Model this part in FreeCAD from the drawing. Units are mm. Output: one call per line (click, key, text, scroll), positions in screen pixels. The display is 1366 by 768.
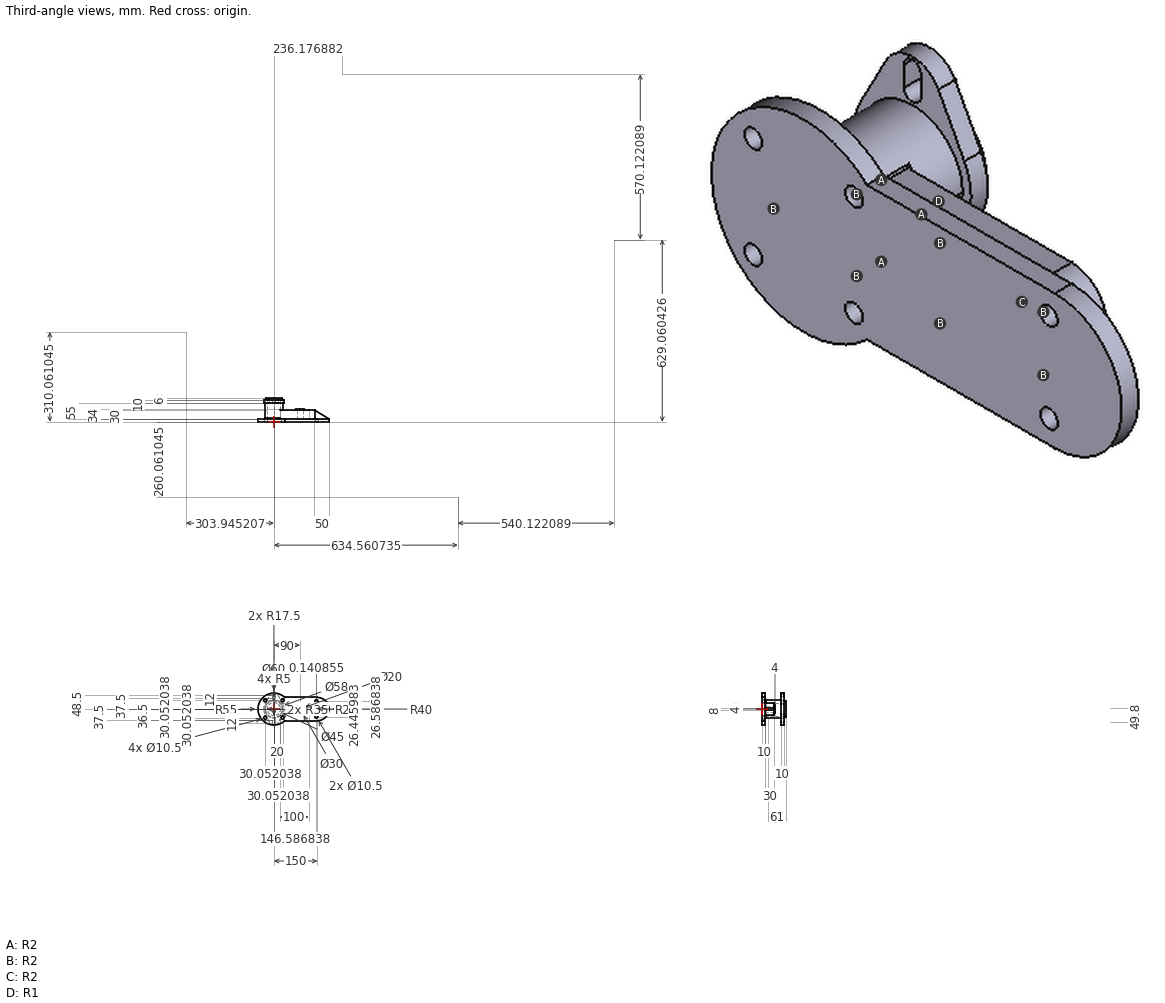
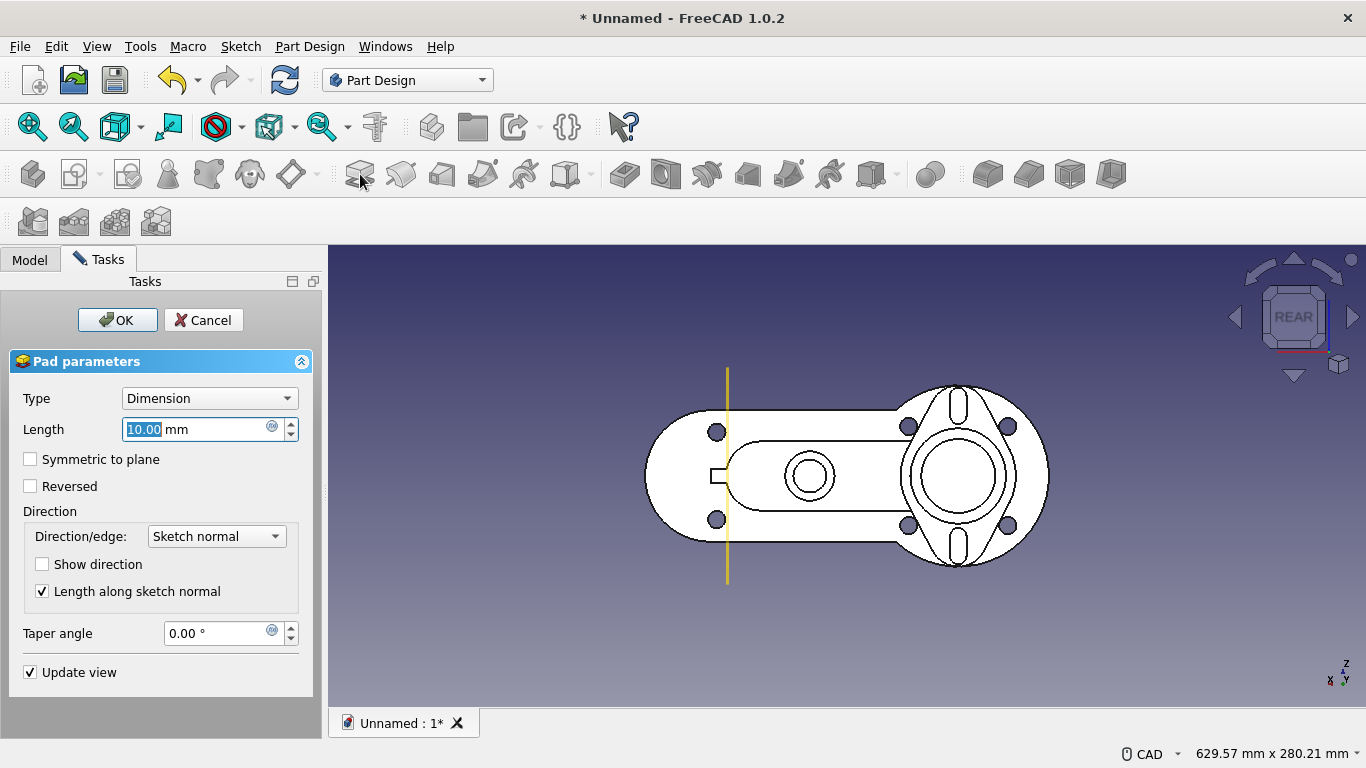
text(50)
key(Tab)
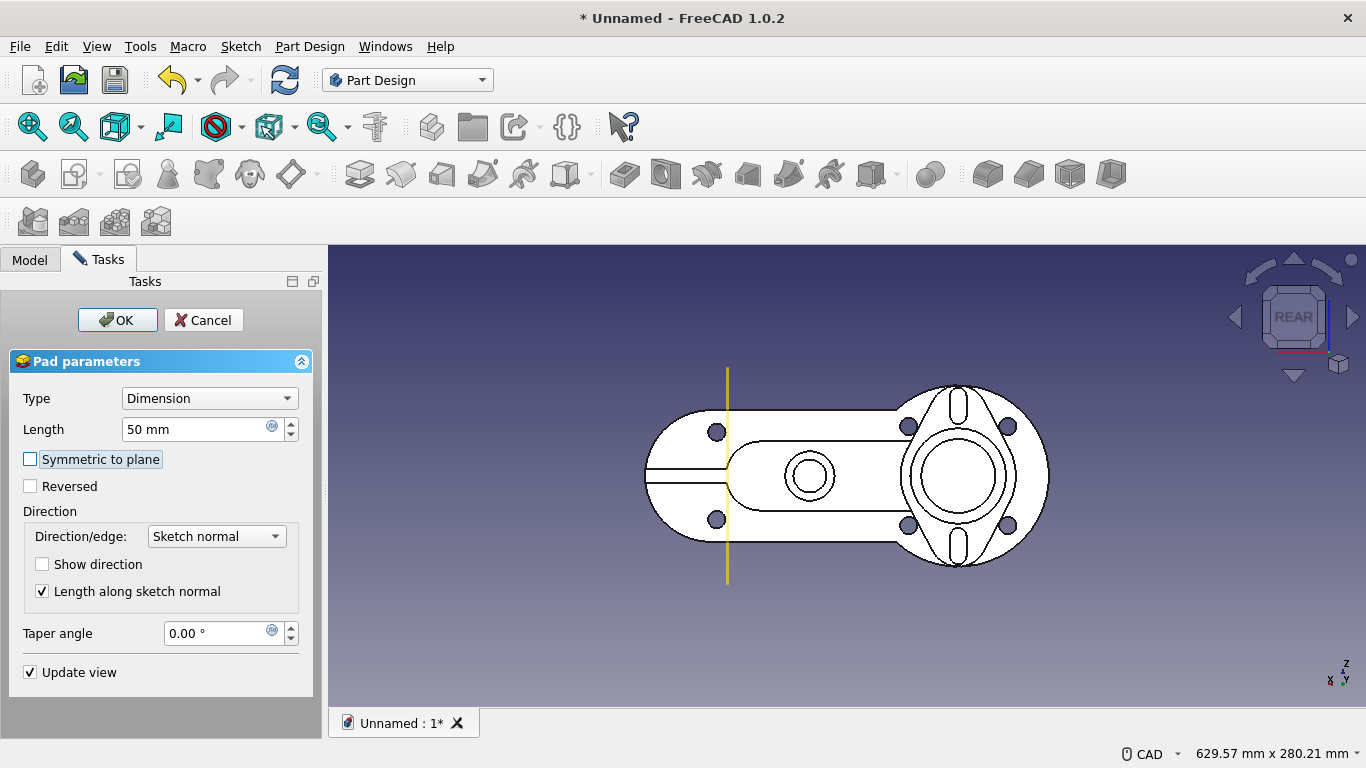
click(118, 320)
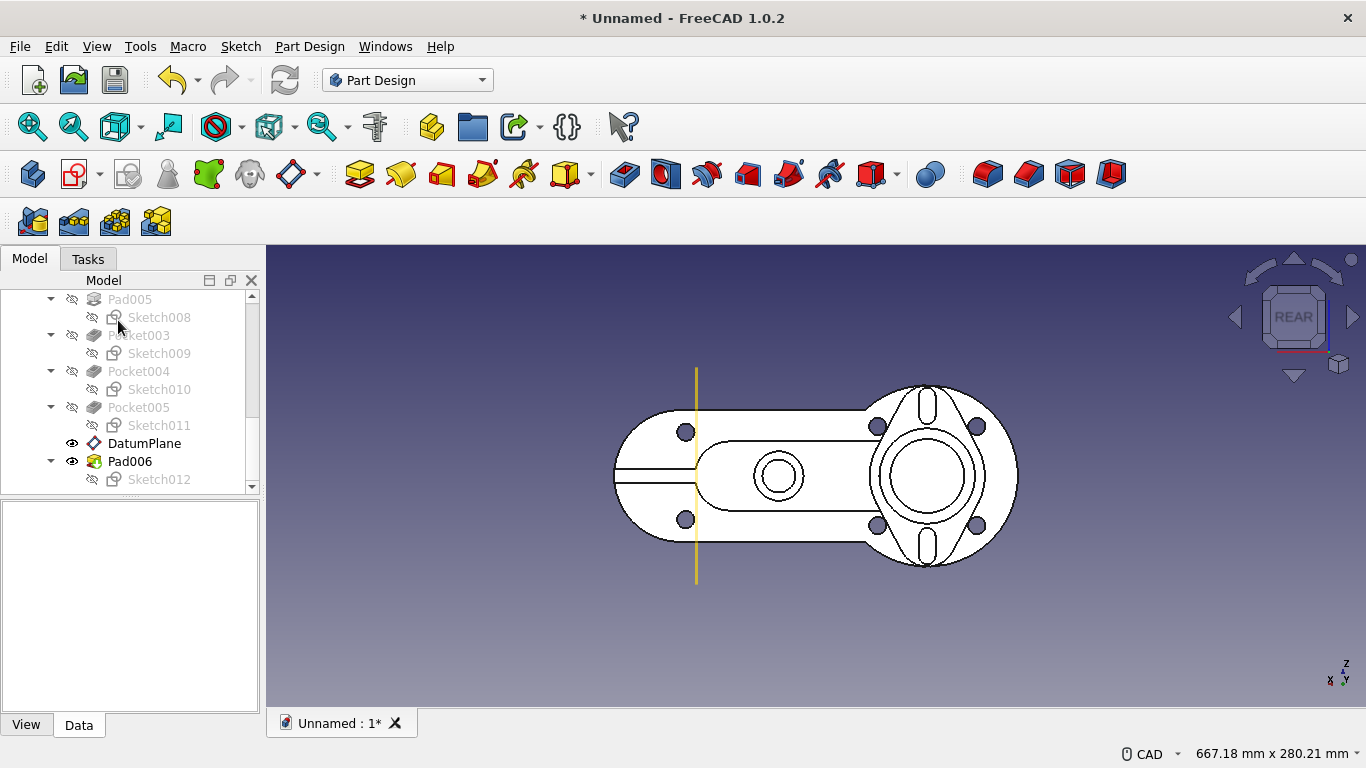
click(117, 443)
key(space)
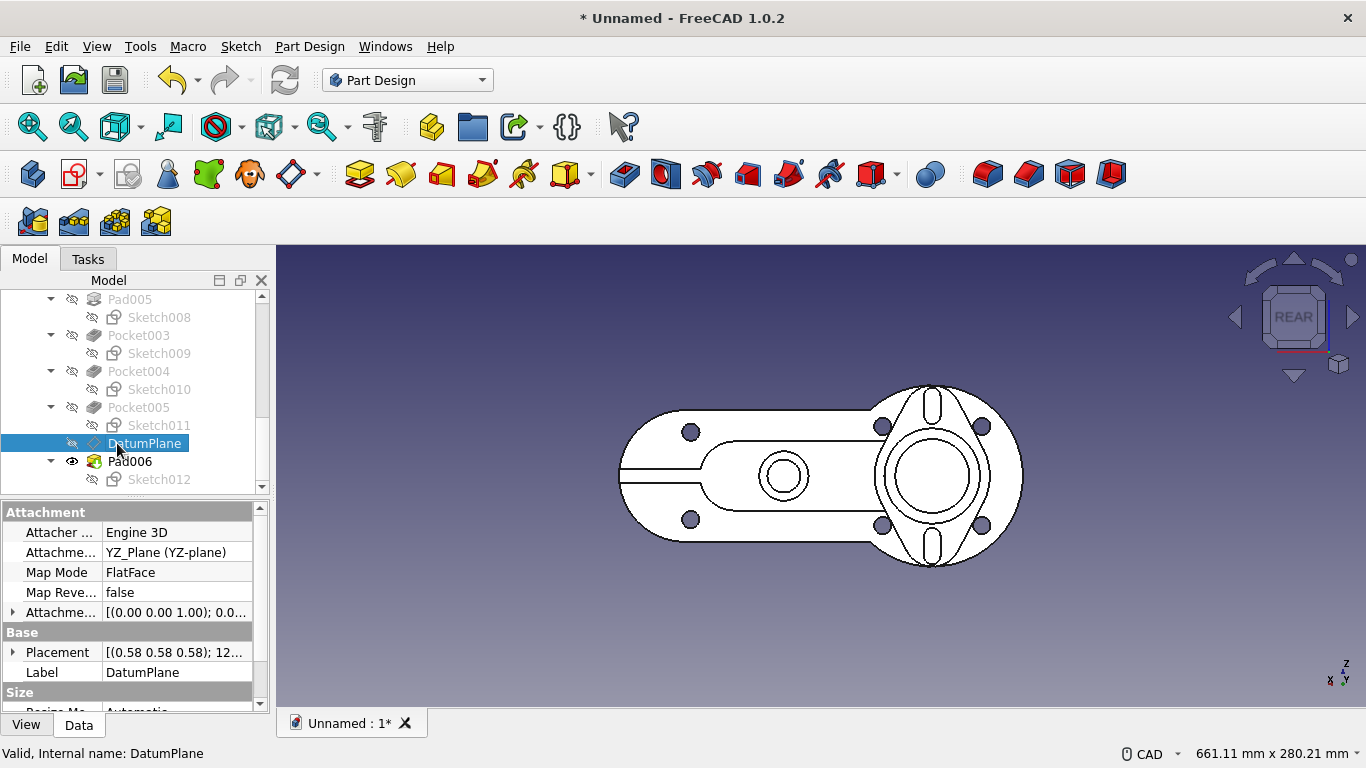
click(33, 128)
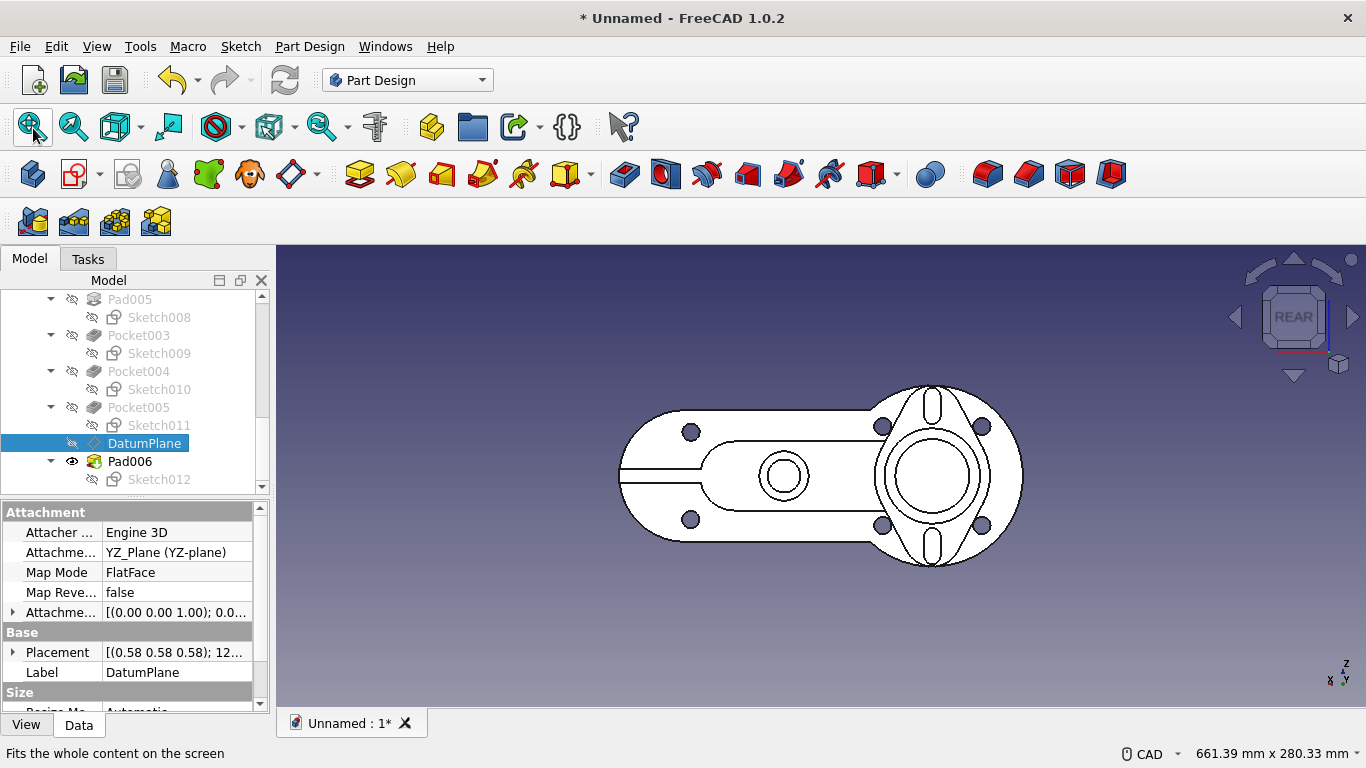
key(0)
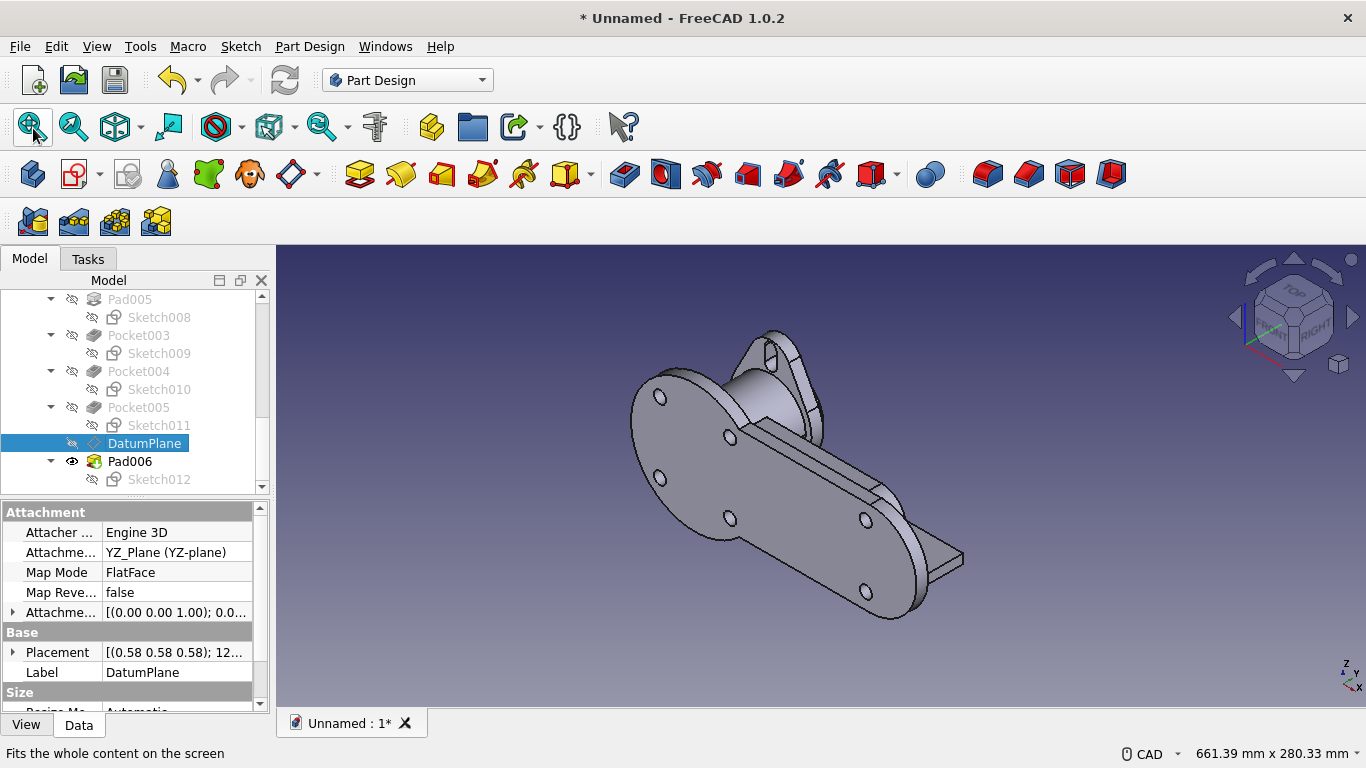
key(2)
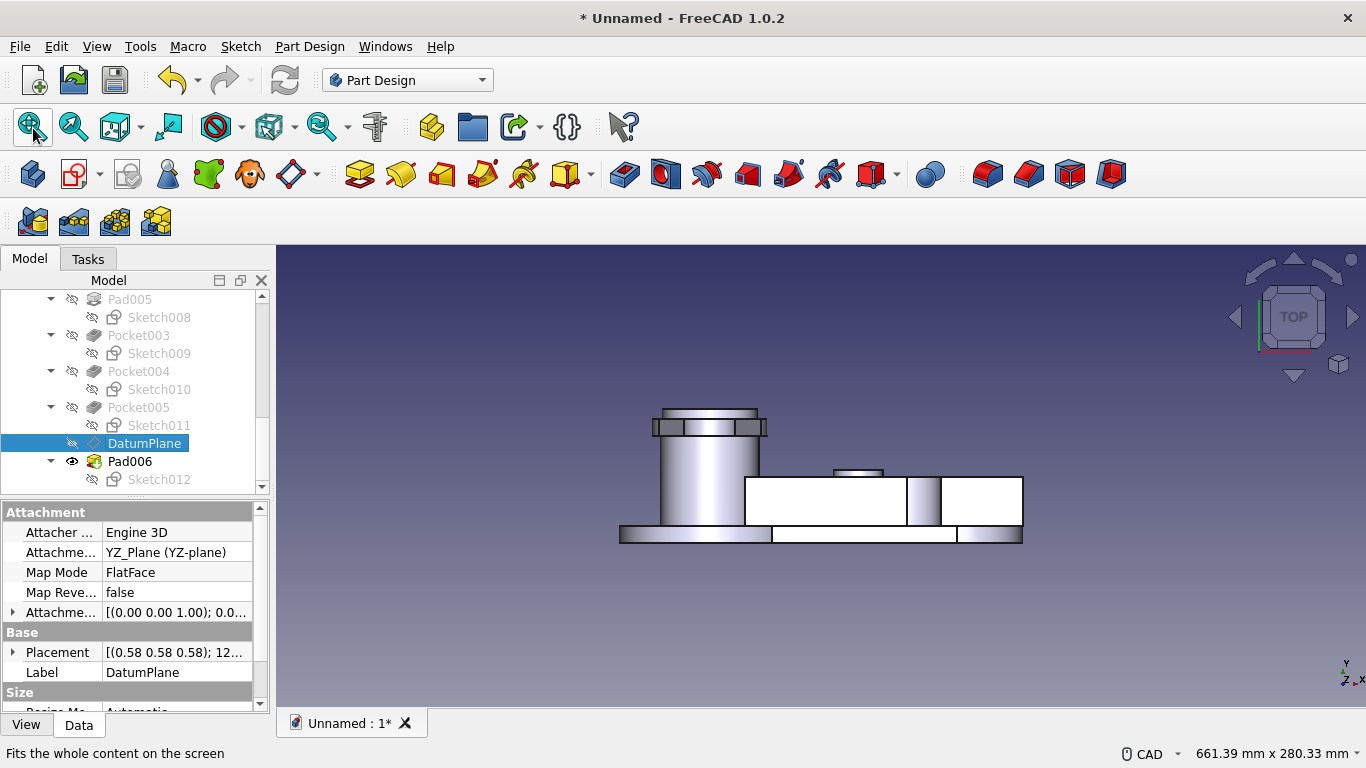
click(33, 128)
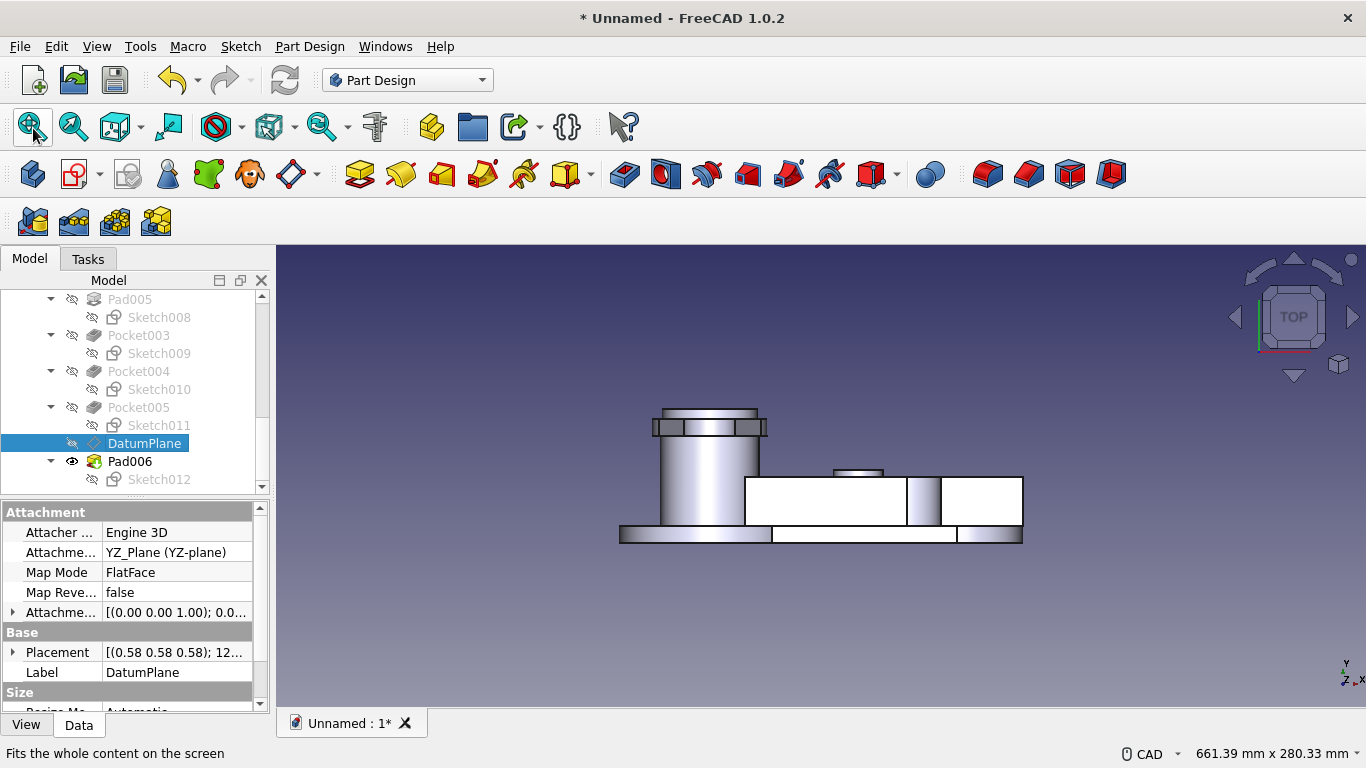
click(994, 501)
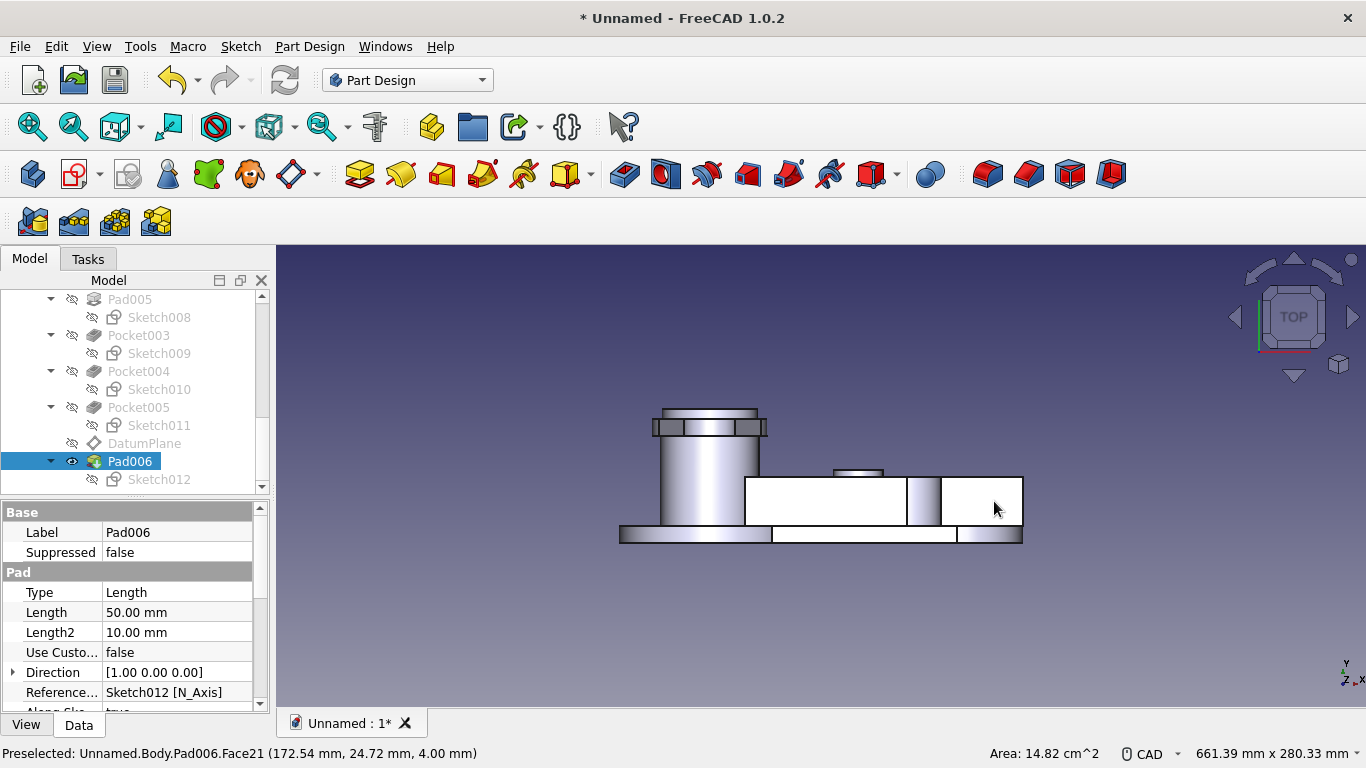
click(74, 174)